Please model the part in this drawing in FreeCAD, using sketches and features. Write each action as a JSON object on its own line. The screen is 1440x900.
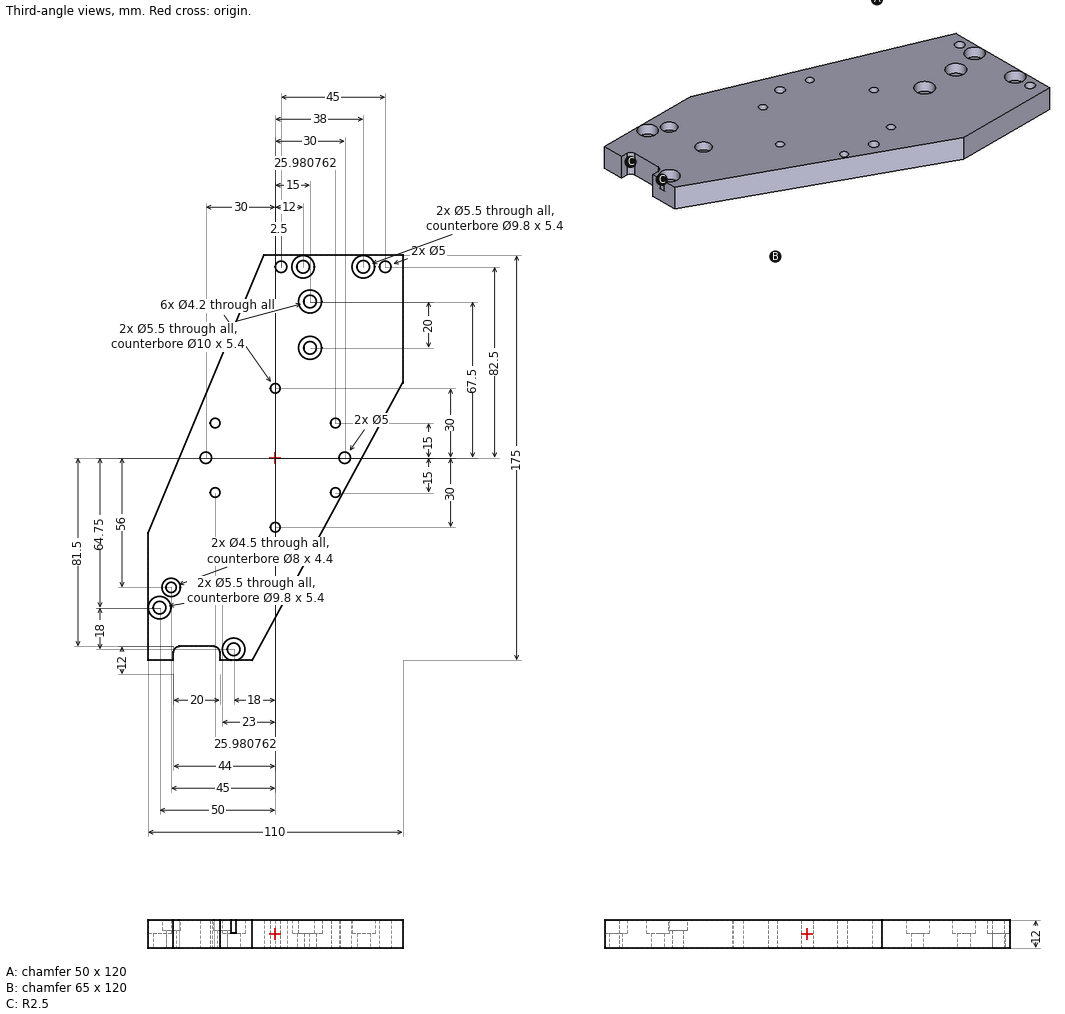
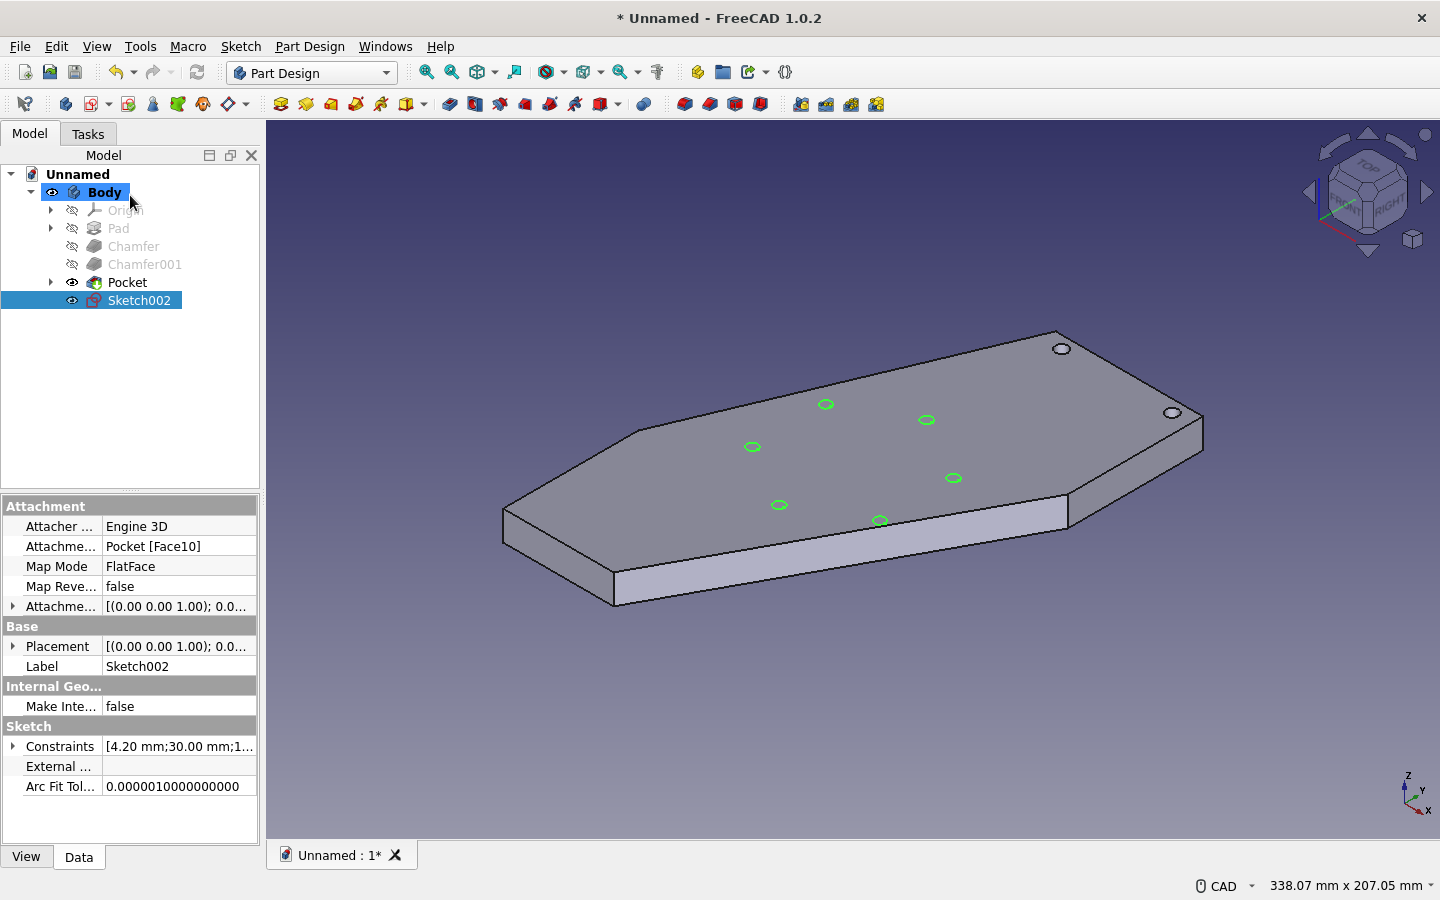
{"action": "left_click", "coordinate": [475, 104]}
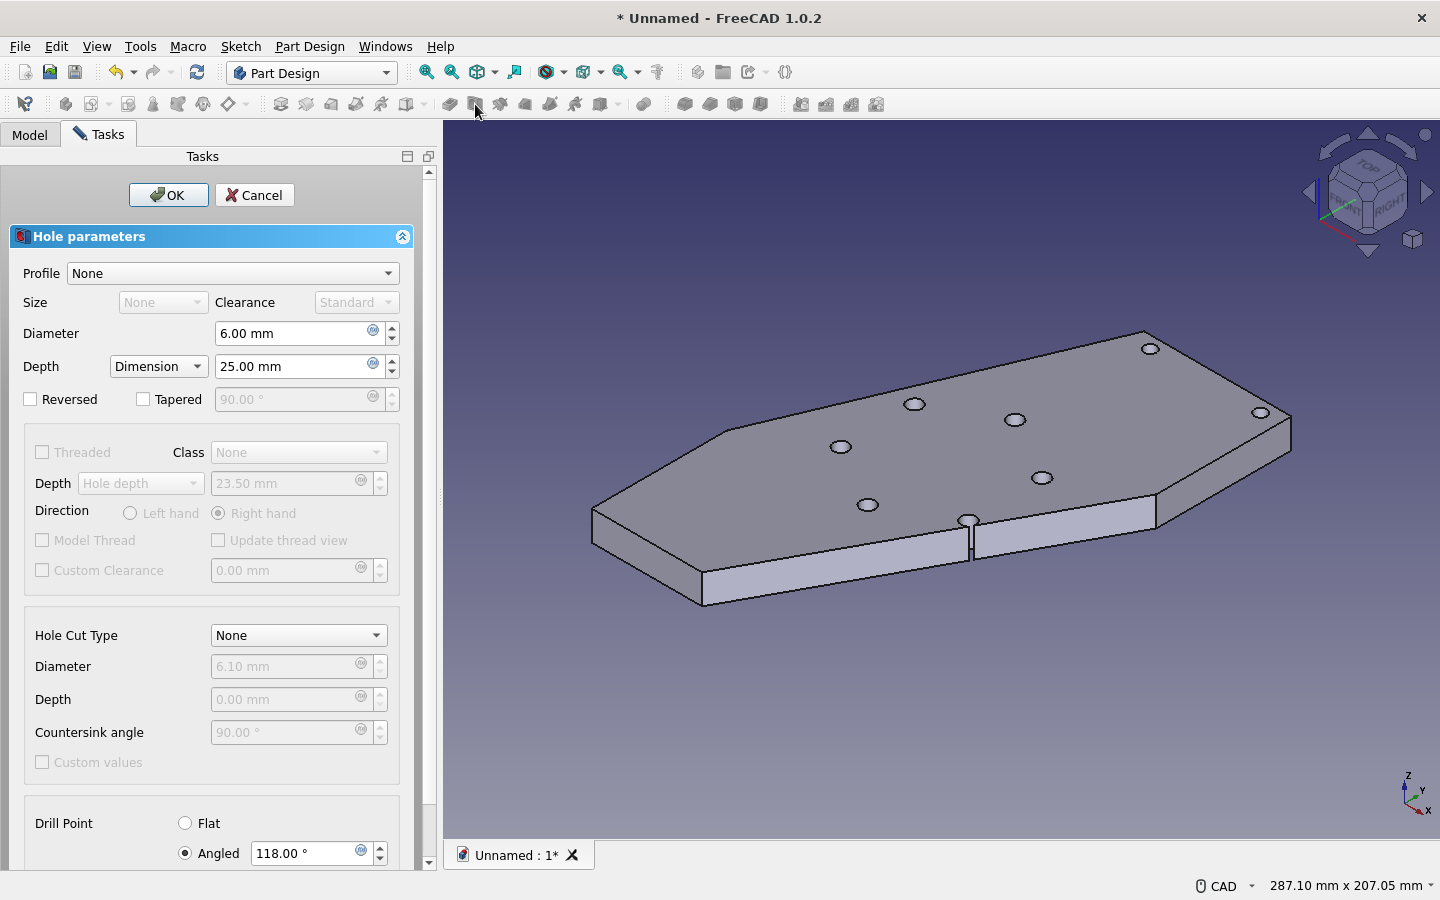
{"action": "triple_click", "coordinate": [300, 334]}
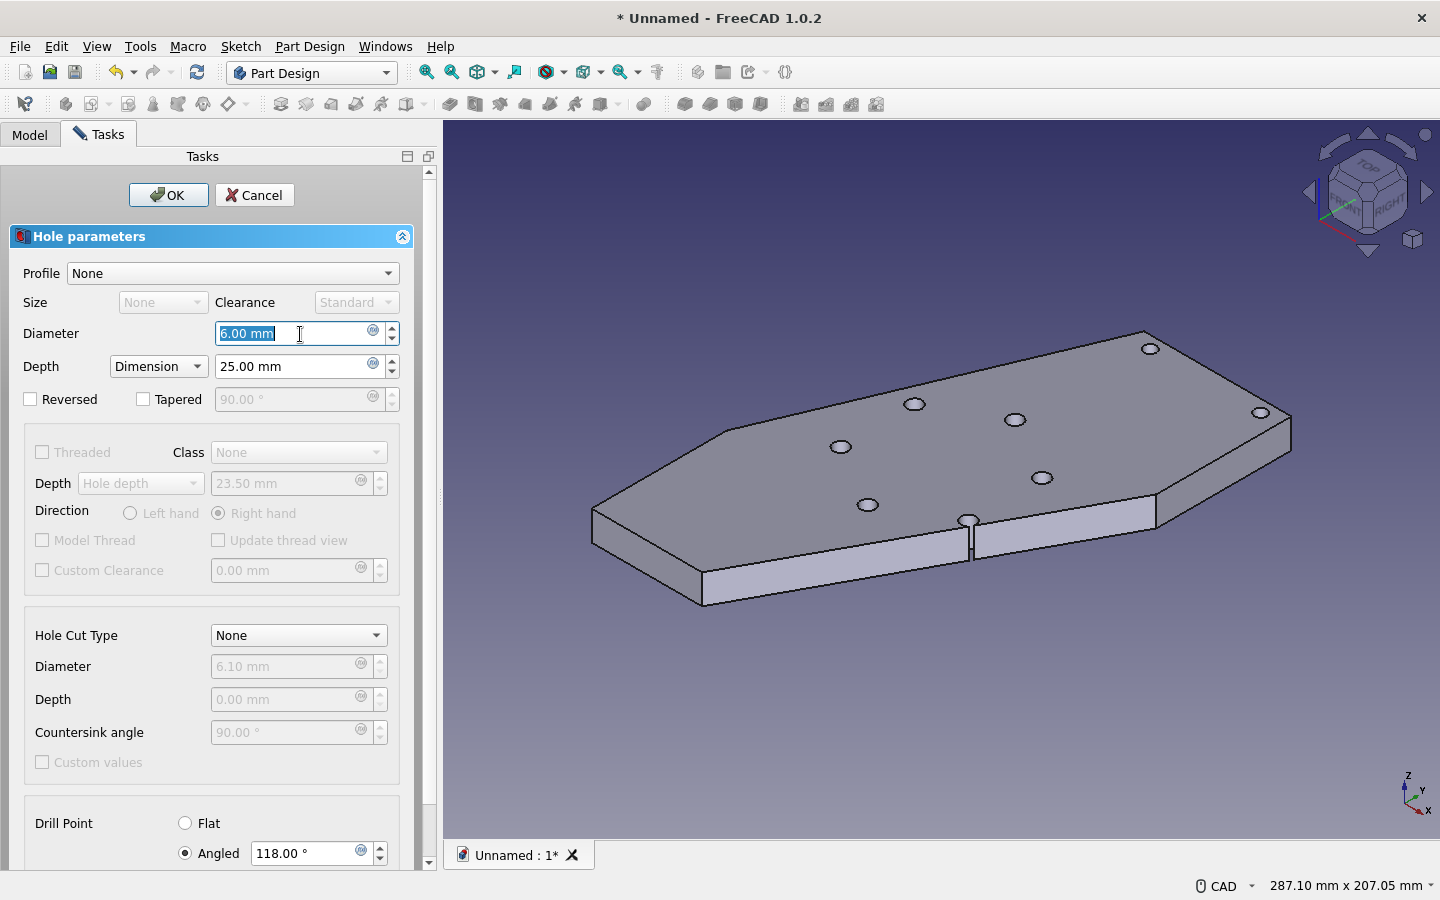
{"action": "type", "text": "4.2"}
{"action": "key", "text": "Tab"}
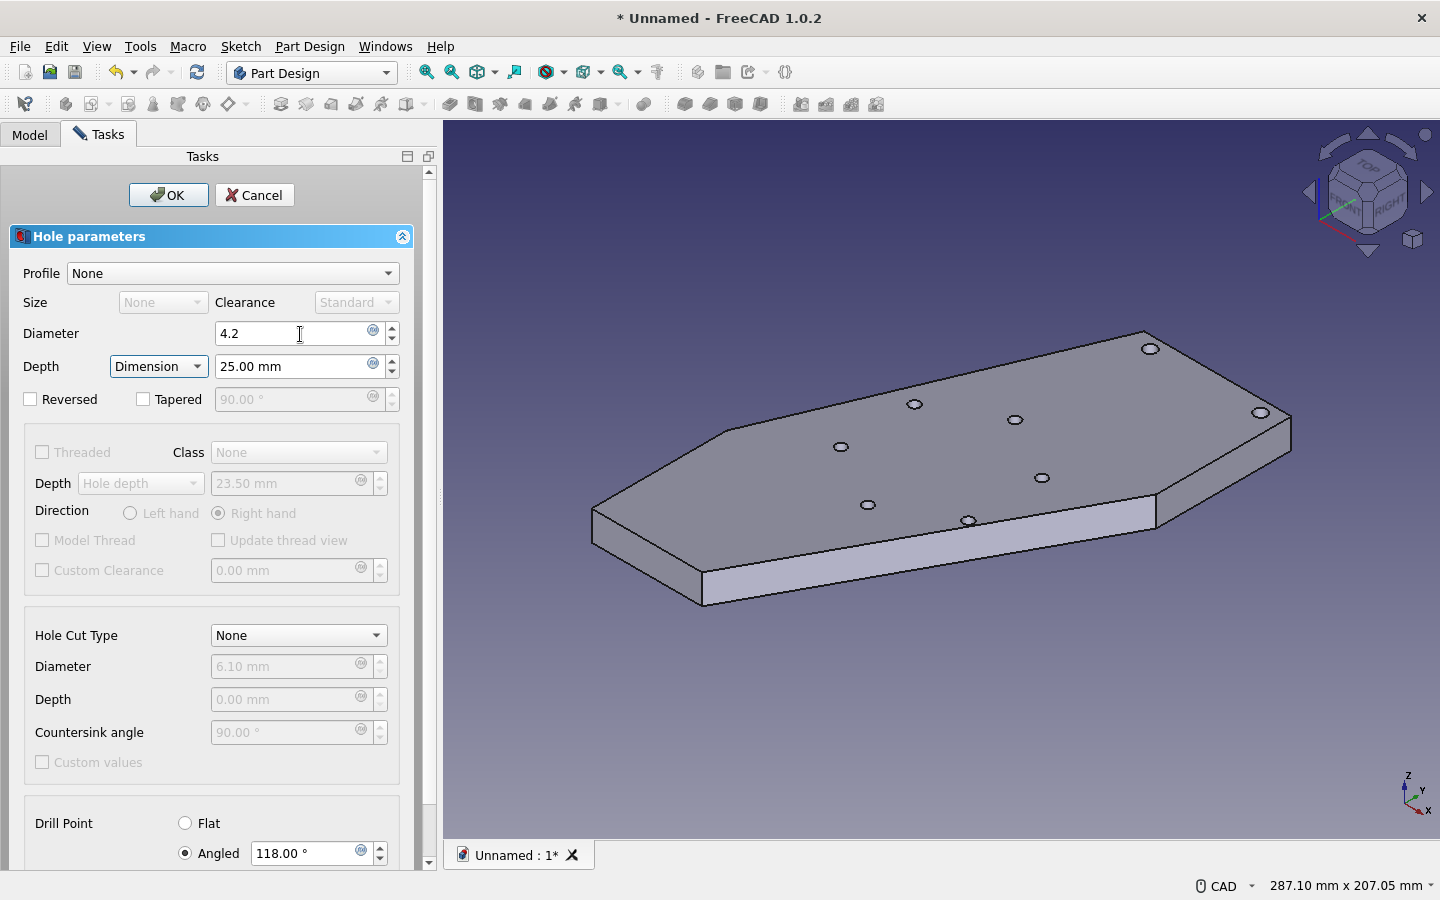
{"action": "left_click", "coordinate": [160, 366]}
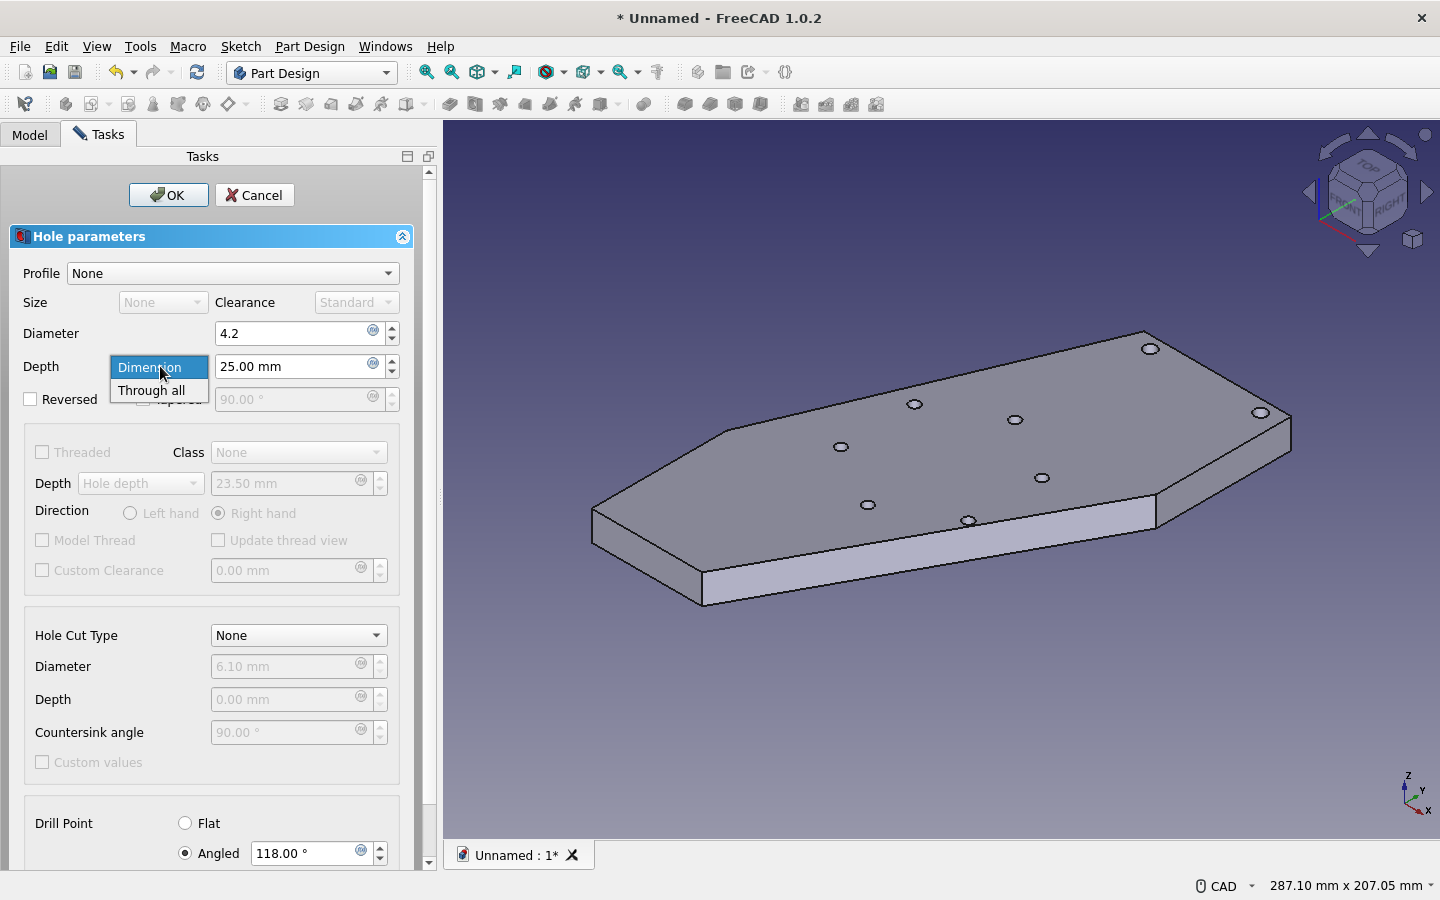
{"action": "left_click", "coordinate": [158, 390]}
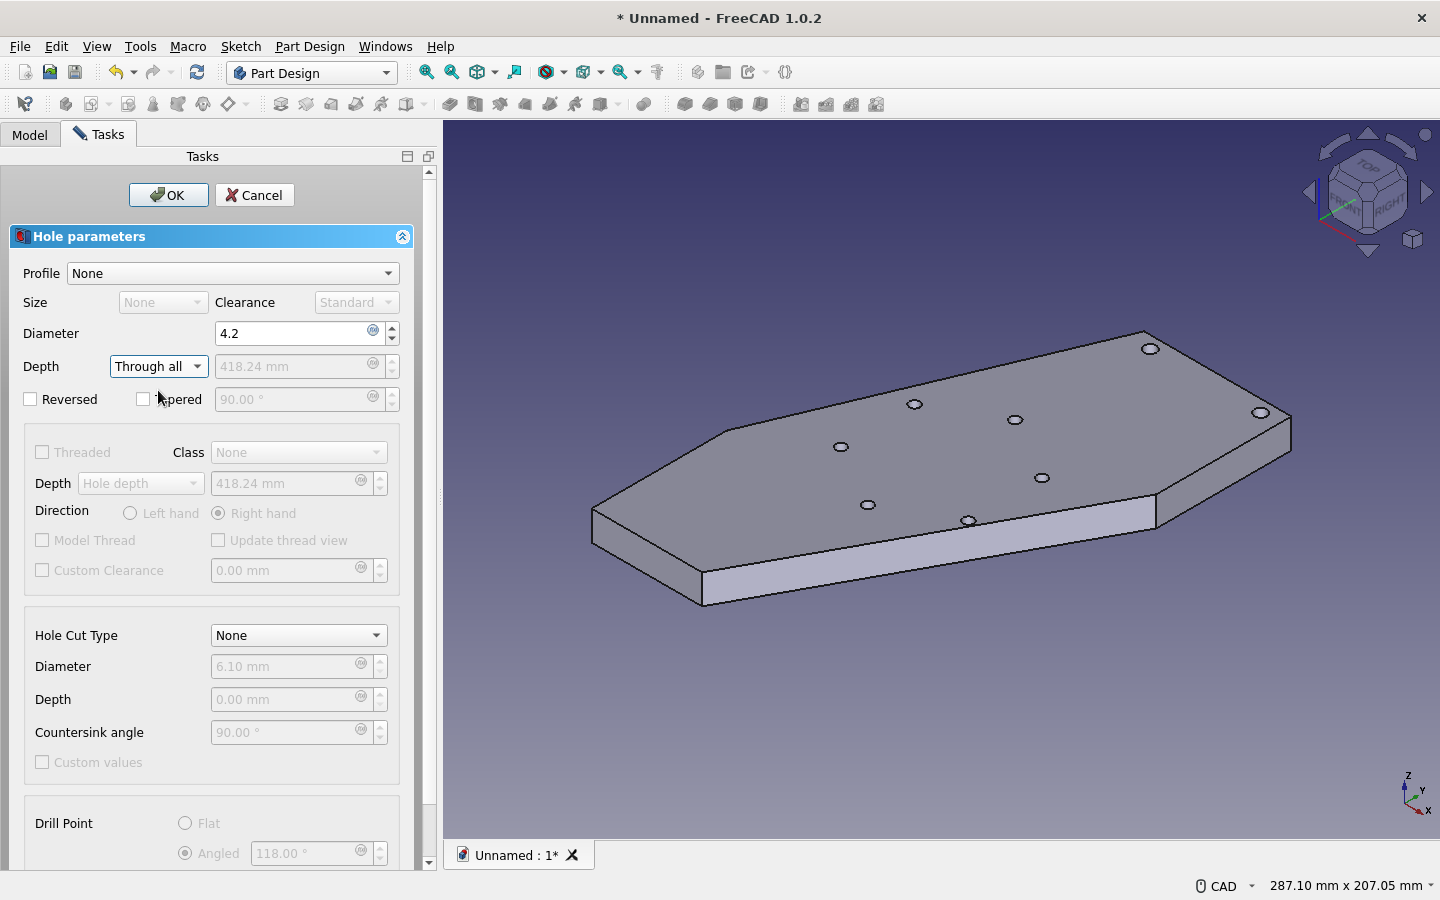
{"action": "left_click", "coordinate": [169, 195]}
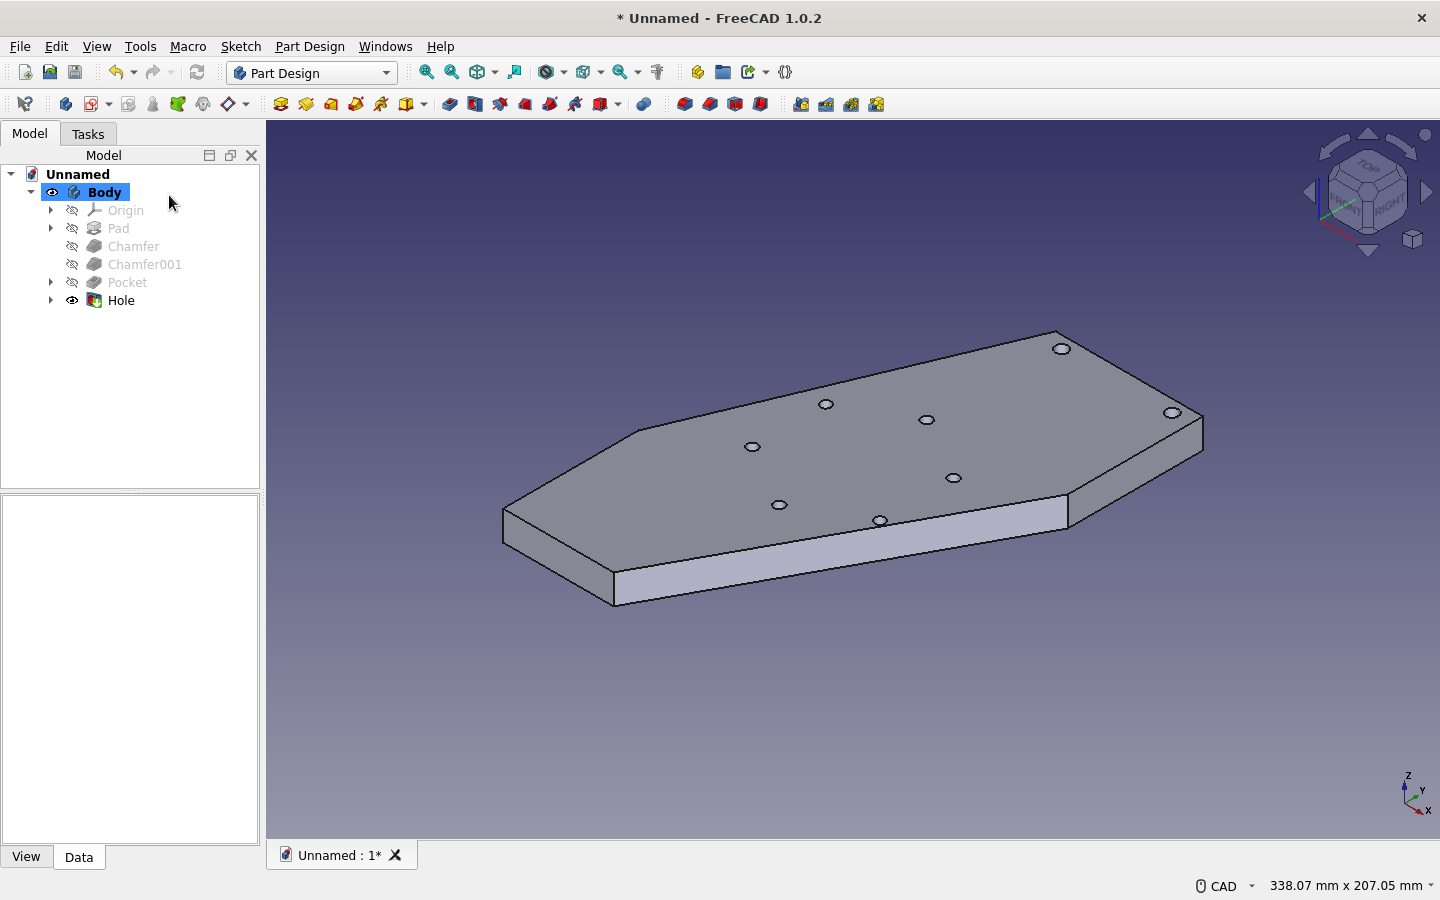
{"action": "left_click", "coordinate": [853, 461]}